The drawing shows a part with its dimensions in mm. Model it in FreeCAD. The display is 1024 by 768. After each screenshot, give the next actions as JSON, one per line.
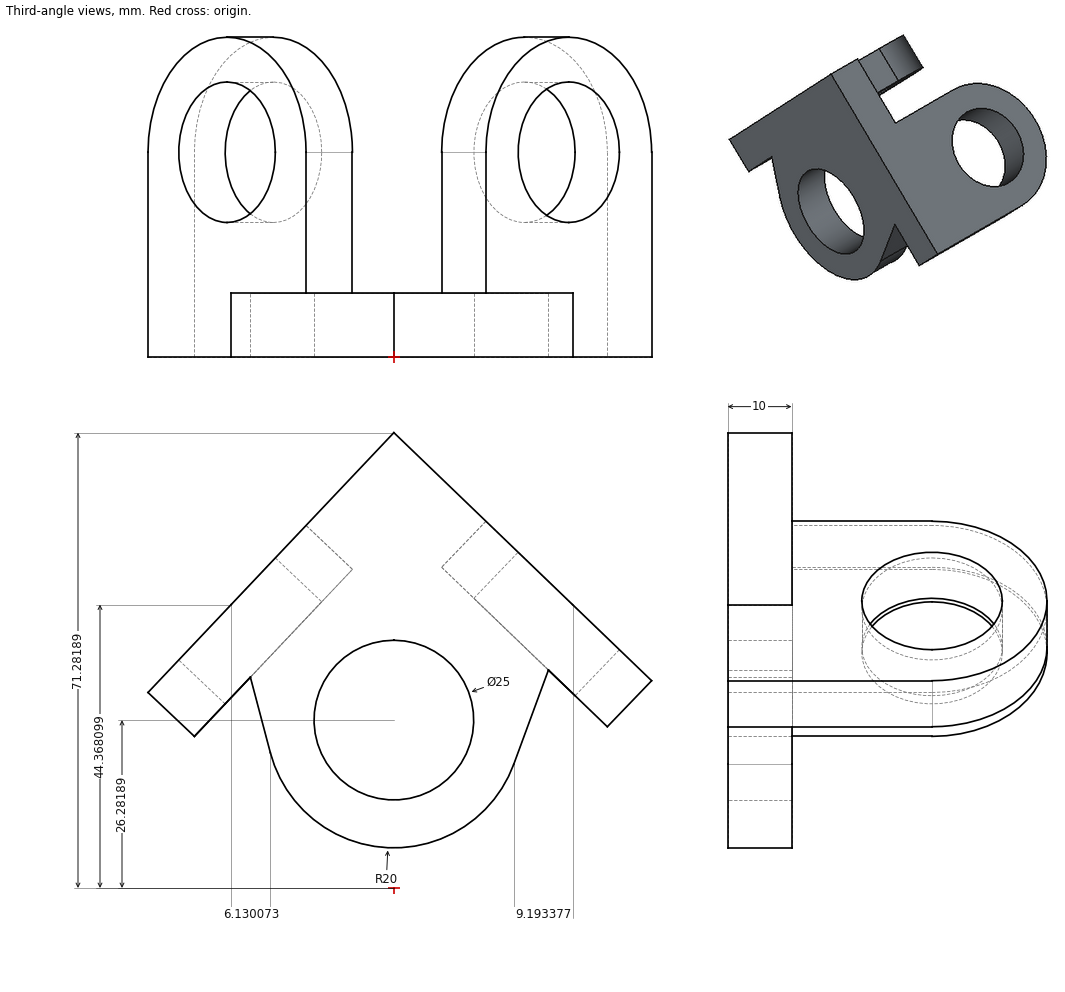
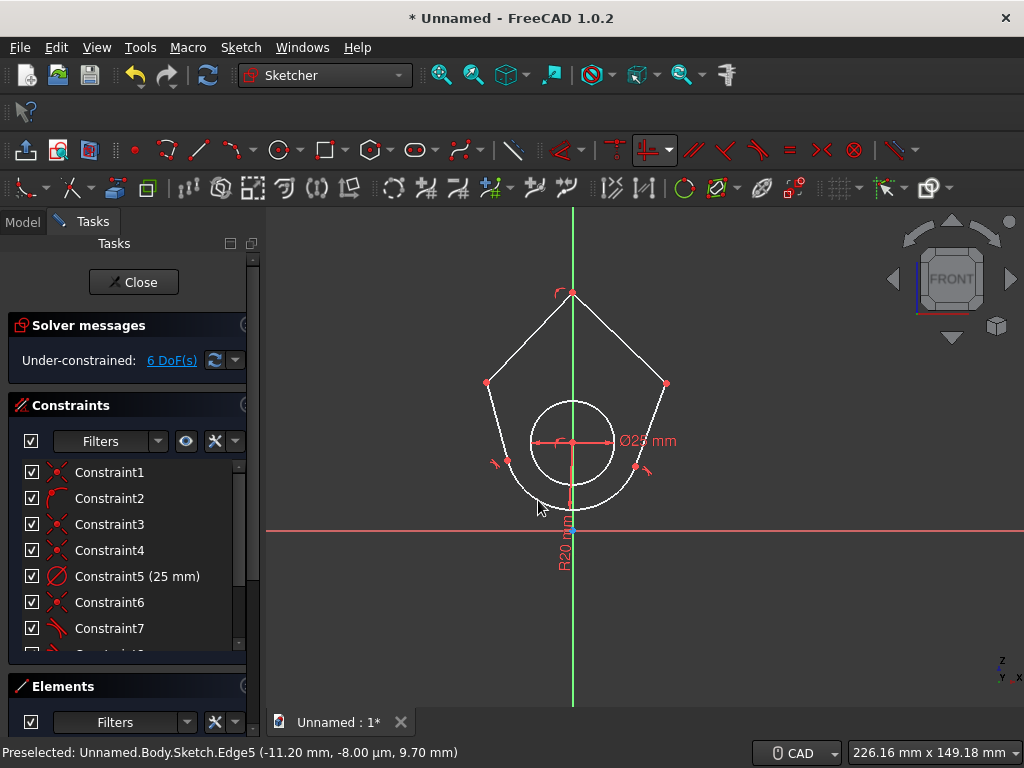
{"action": "left_click", "coordinate": [573, 443]}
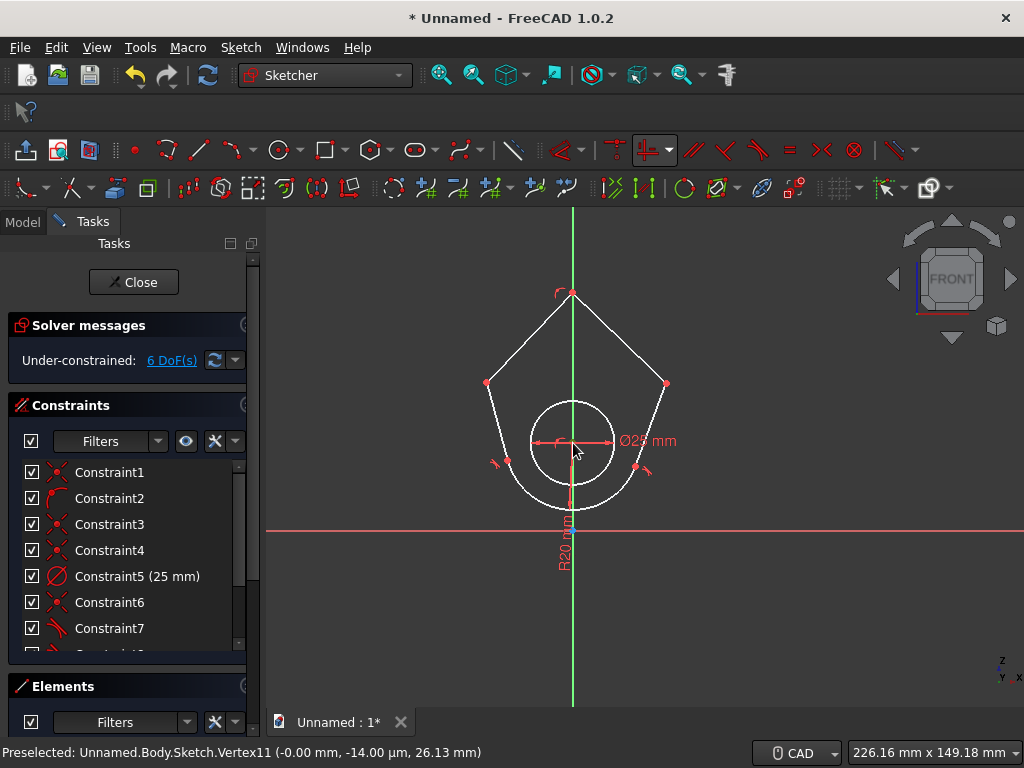
{"action": "left_click", "coordinate": [584, 150]}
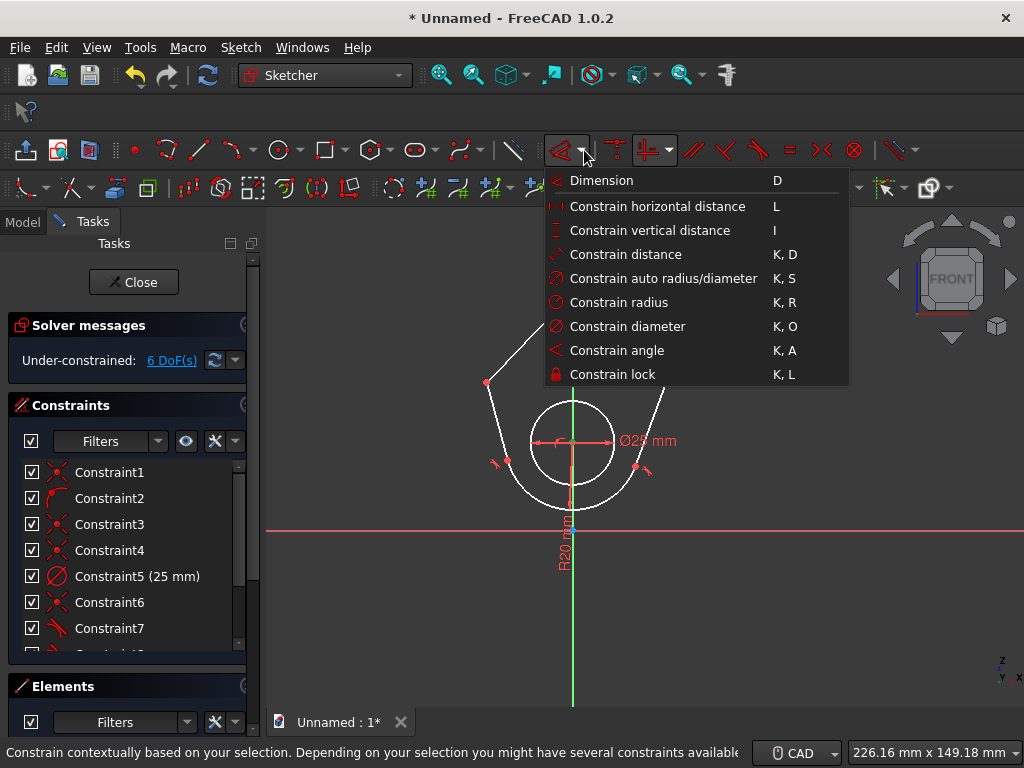
{"action": "left_click", "coordinate": [697, 230]}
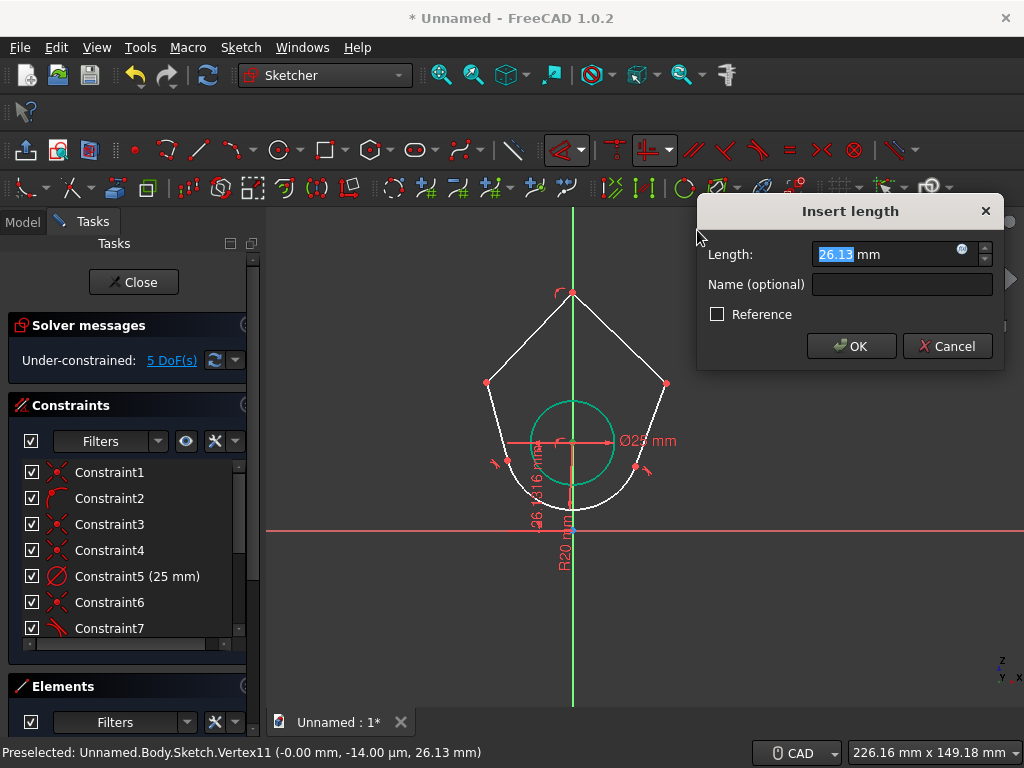
{"action": "type", "text": "26.28189"}
{"action": "key", "text": "Return"}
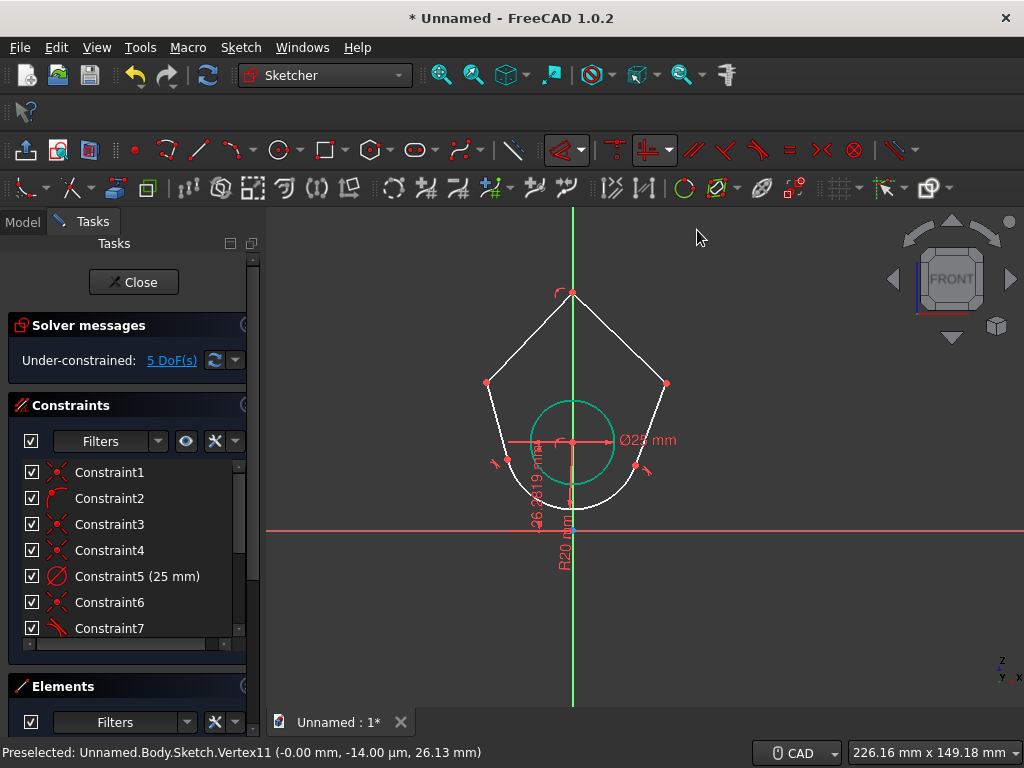
{"action": "left_click", "coordinate": [573, 293]}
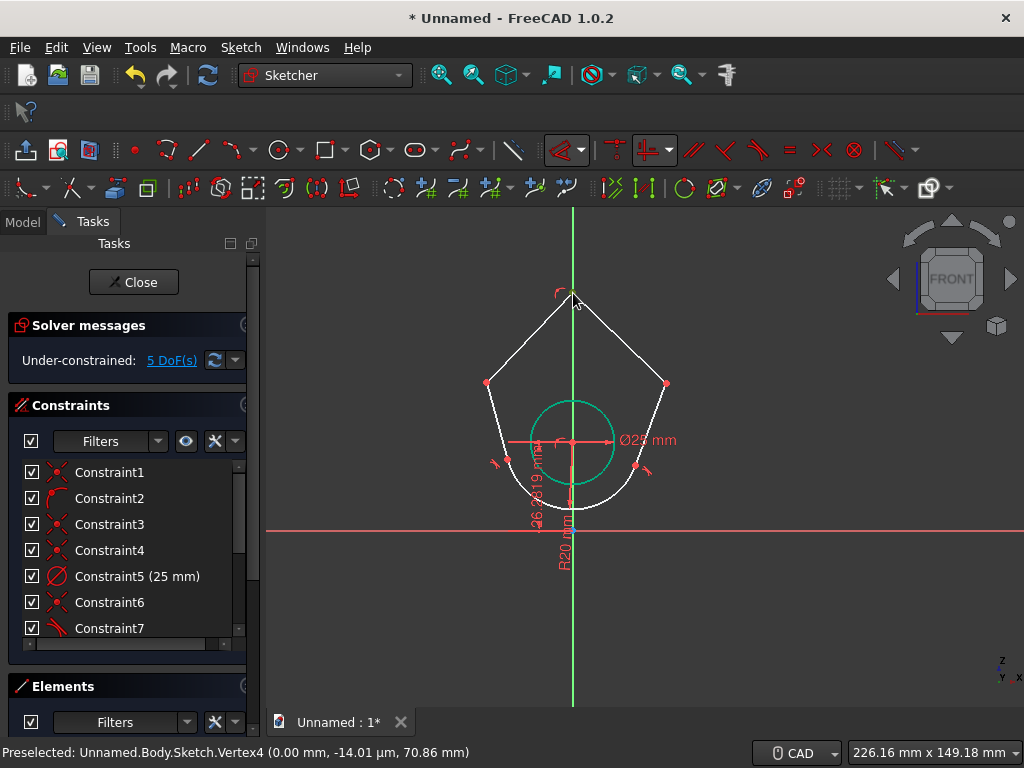
{"action": "left_click", "coordinate": [584, 150]}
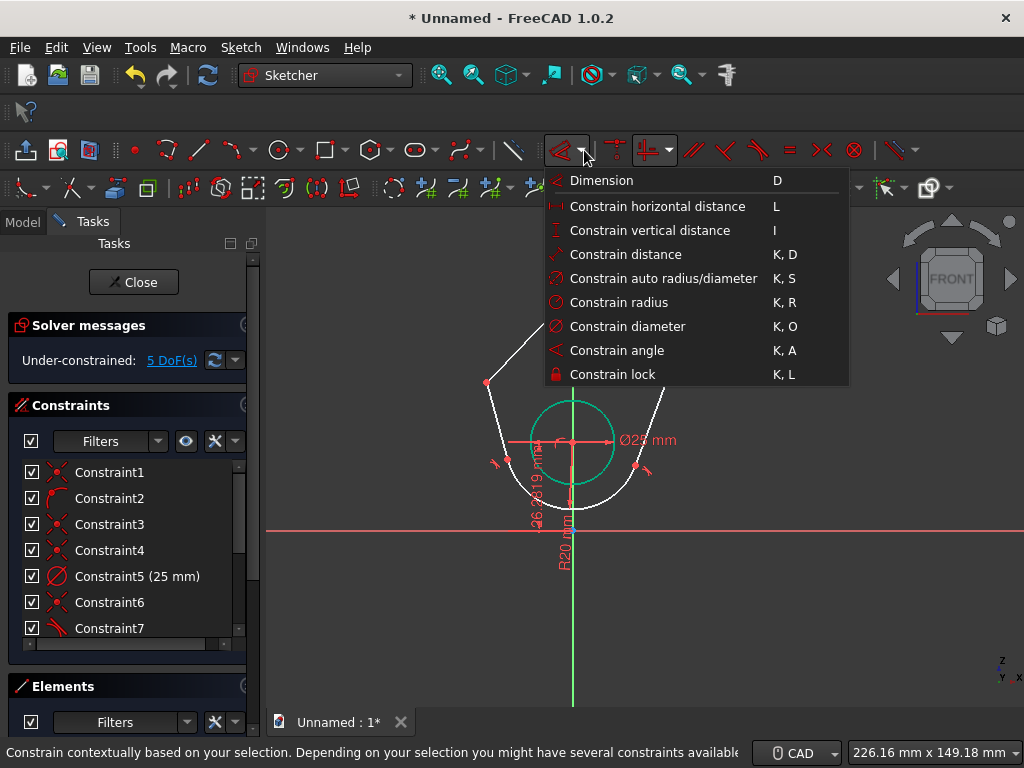
{"action": "left_click", "coordinate": [697, 230]}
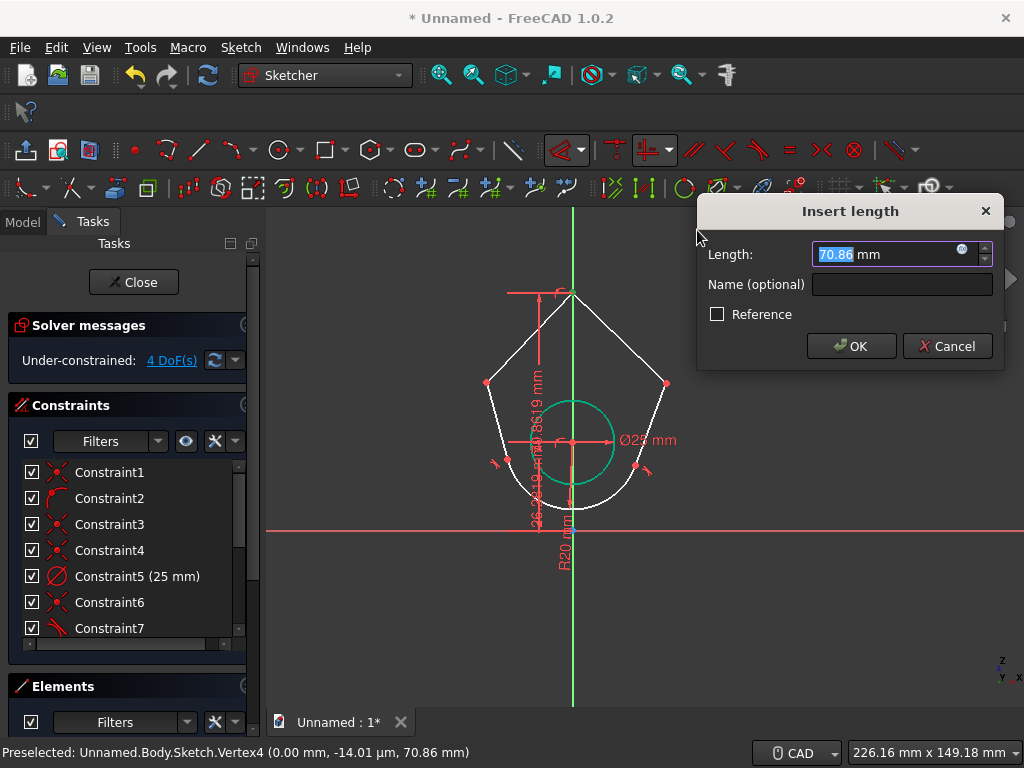
{"action": "type", "text": "71.28189"}
{"action": "key", "text": "Return"}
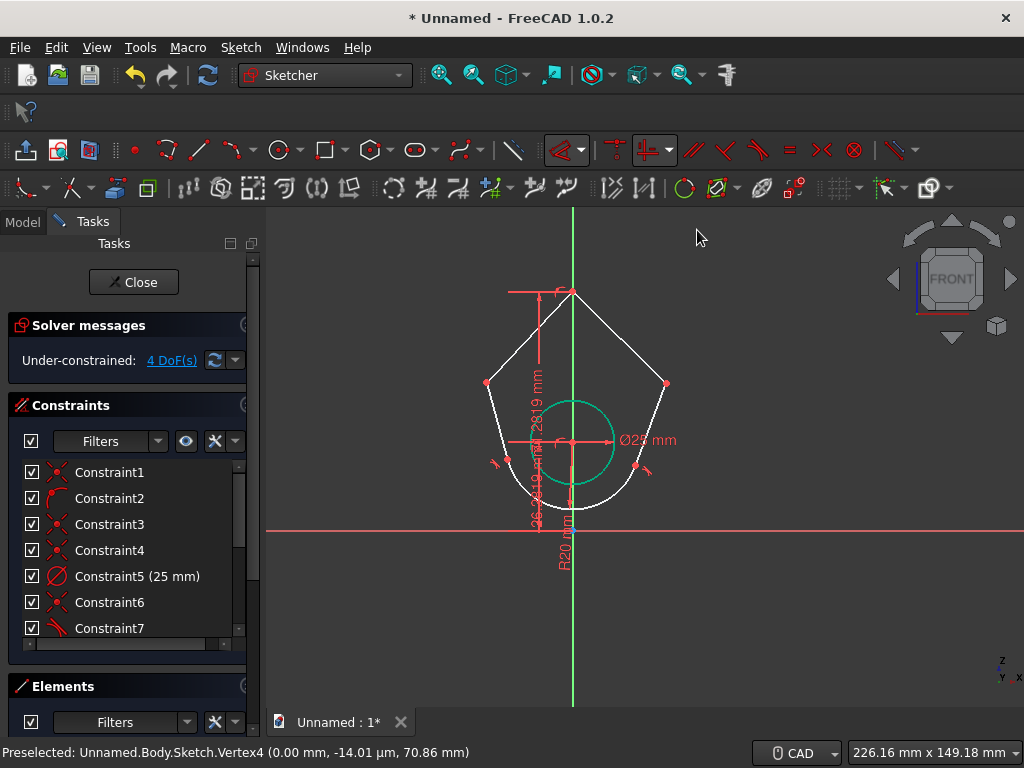
{"action": "scroll", "coordinate": [502, 437], "scroll_direction": "up", "scroll_amount": 4}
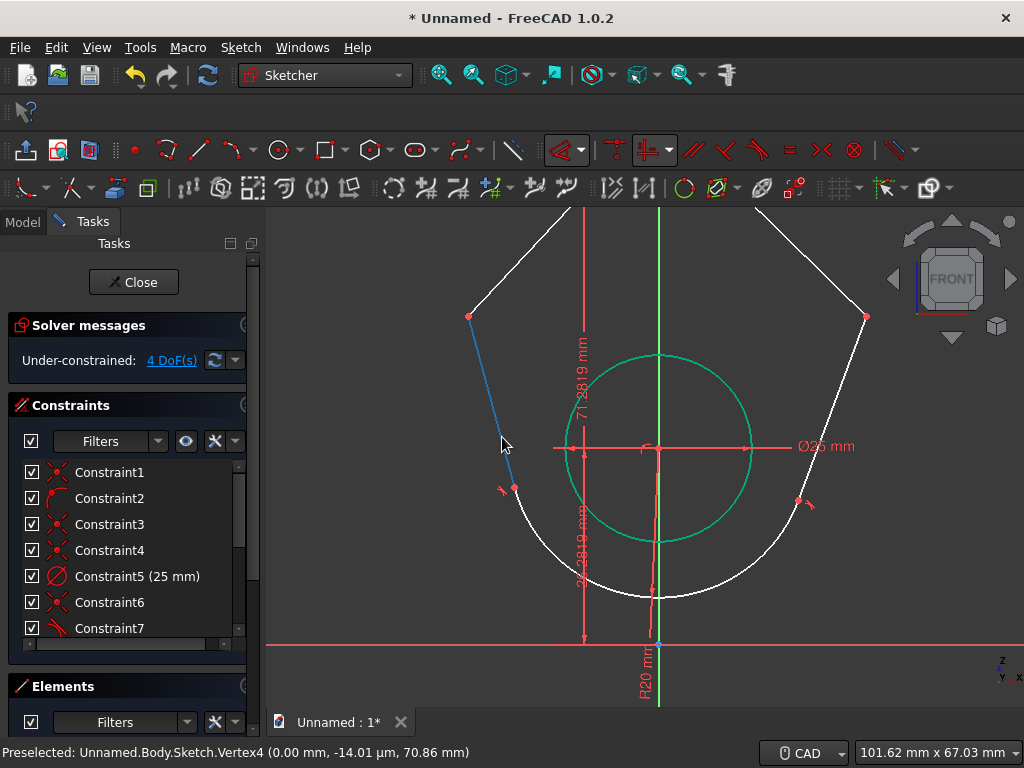
{"action": "left_click", "coordinate": [501, 436]}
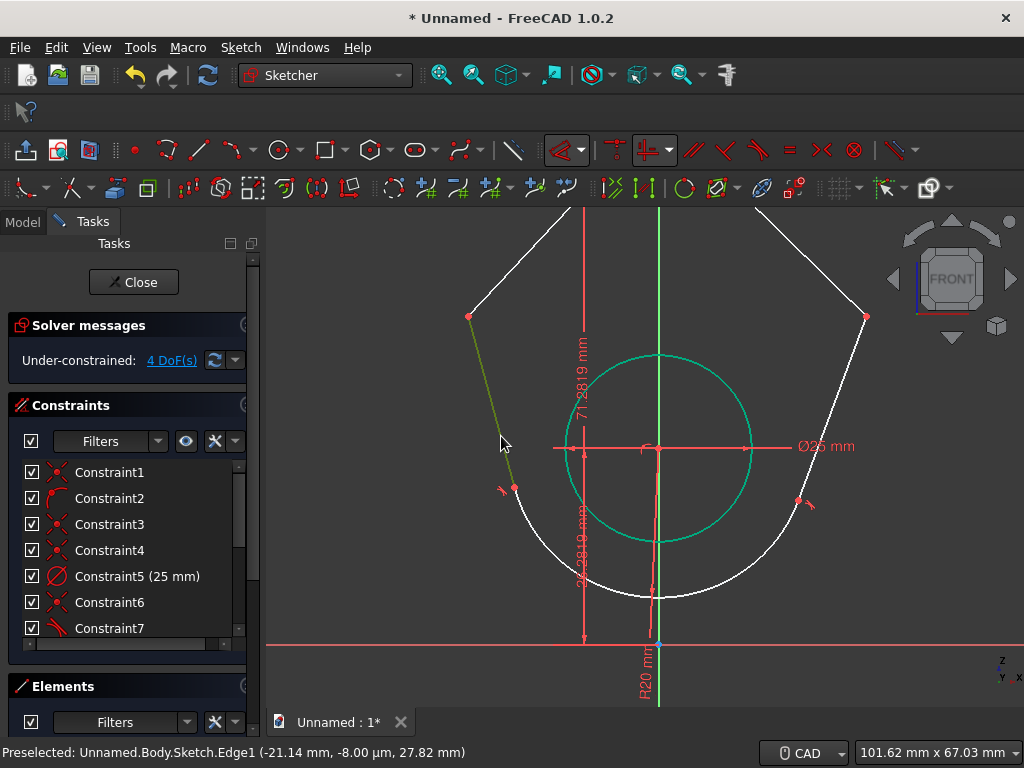
{"action": "left_click", "coordinate": [584, 150]}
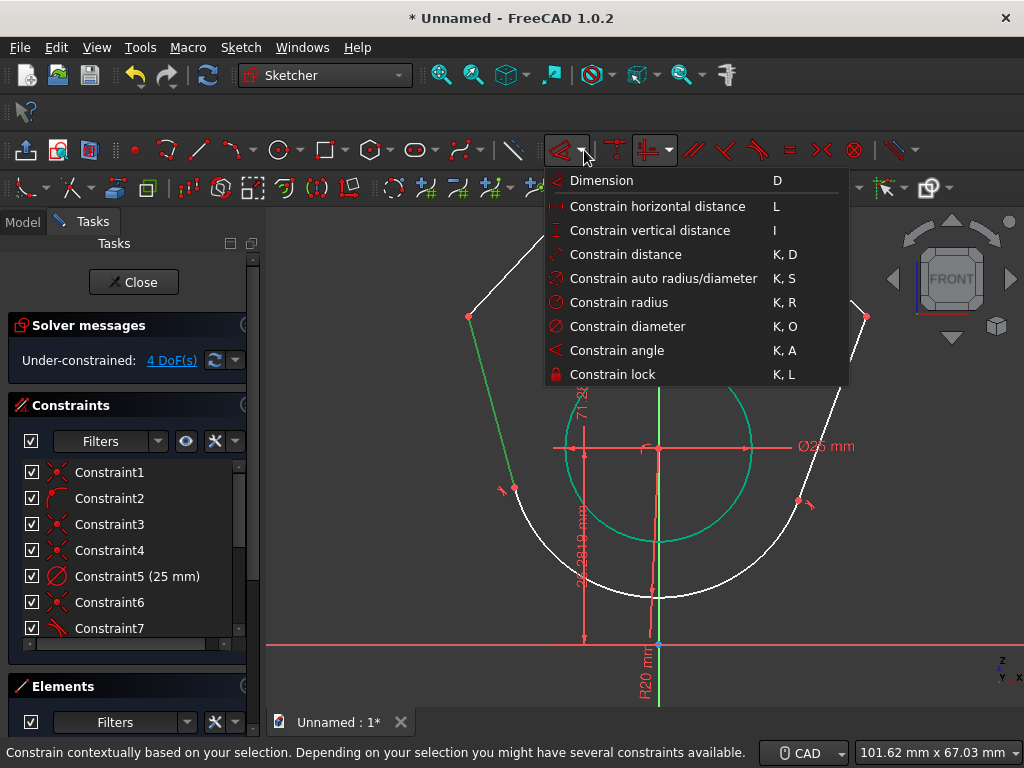
{"action": "left_click", "coordinate": [697, 206]}